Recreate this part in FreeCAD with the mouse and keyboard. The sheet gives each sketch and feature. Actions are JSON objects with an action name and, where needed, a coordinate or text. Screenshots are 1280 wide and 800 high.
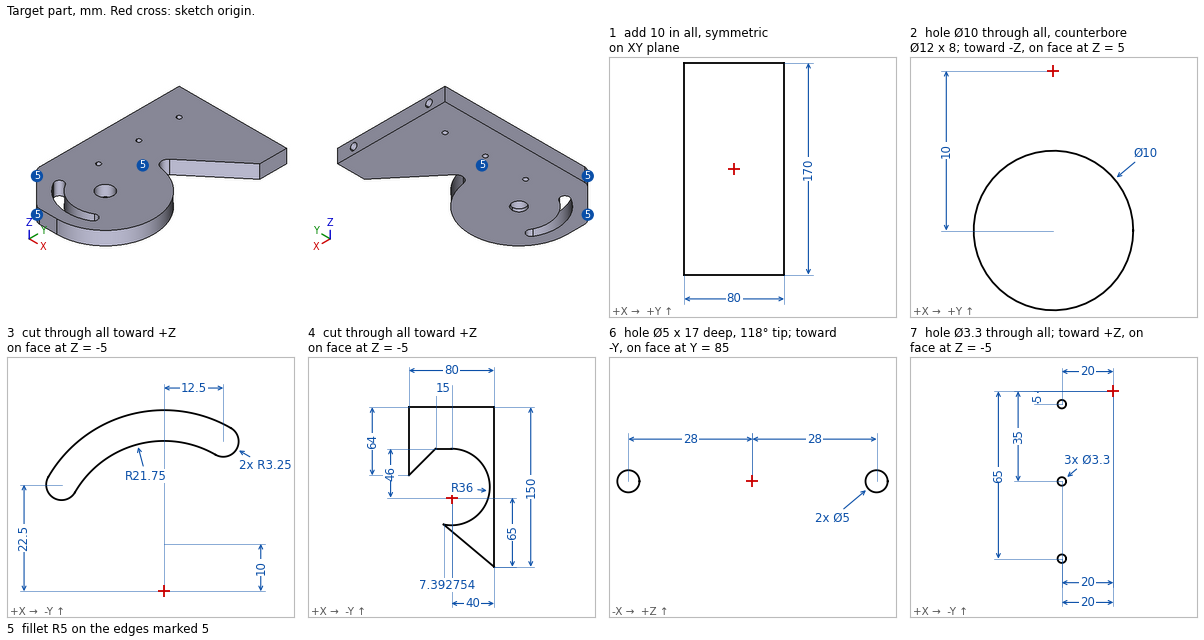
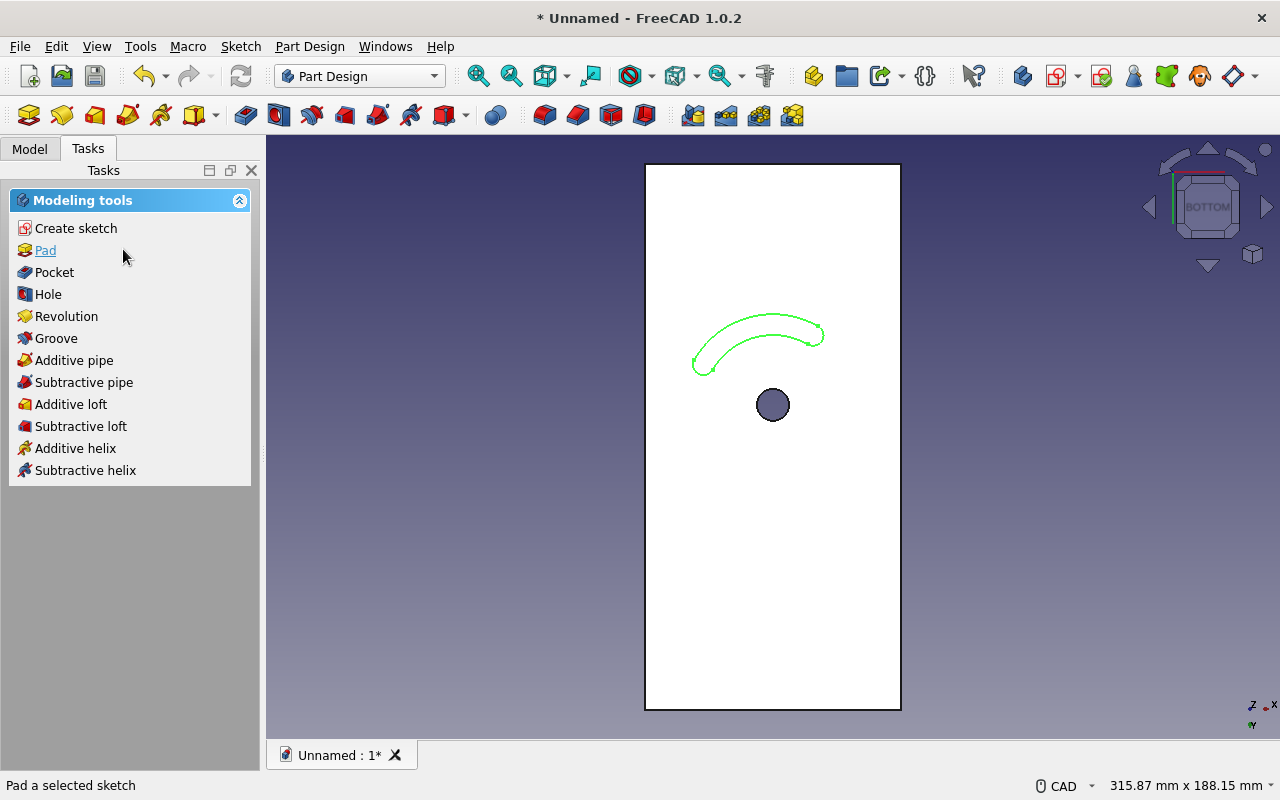
{"action": "left_click", "coordinate": [246, 116]}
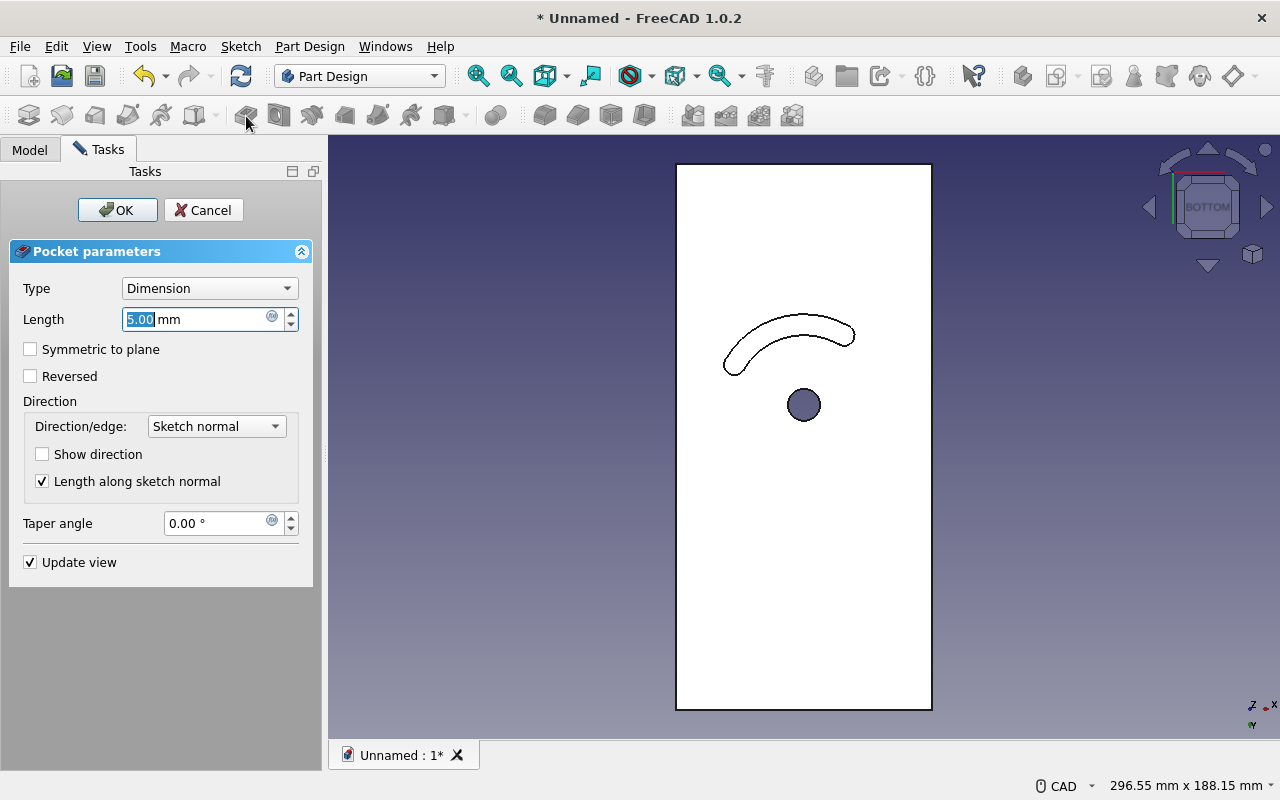
{"action": "left_click", "coordinate": [210, 288]}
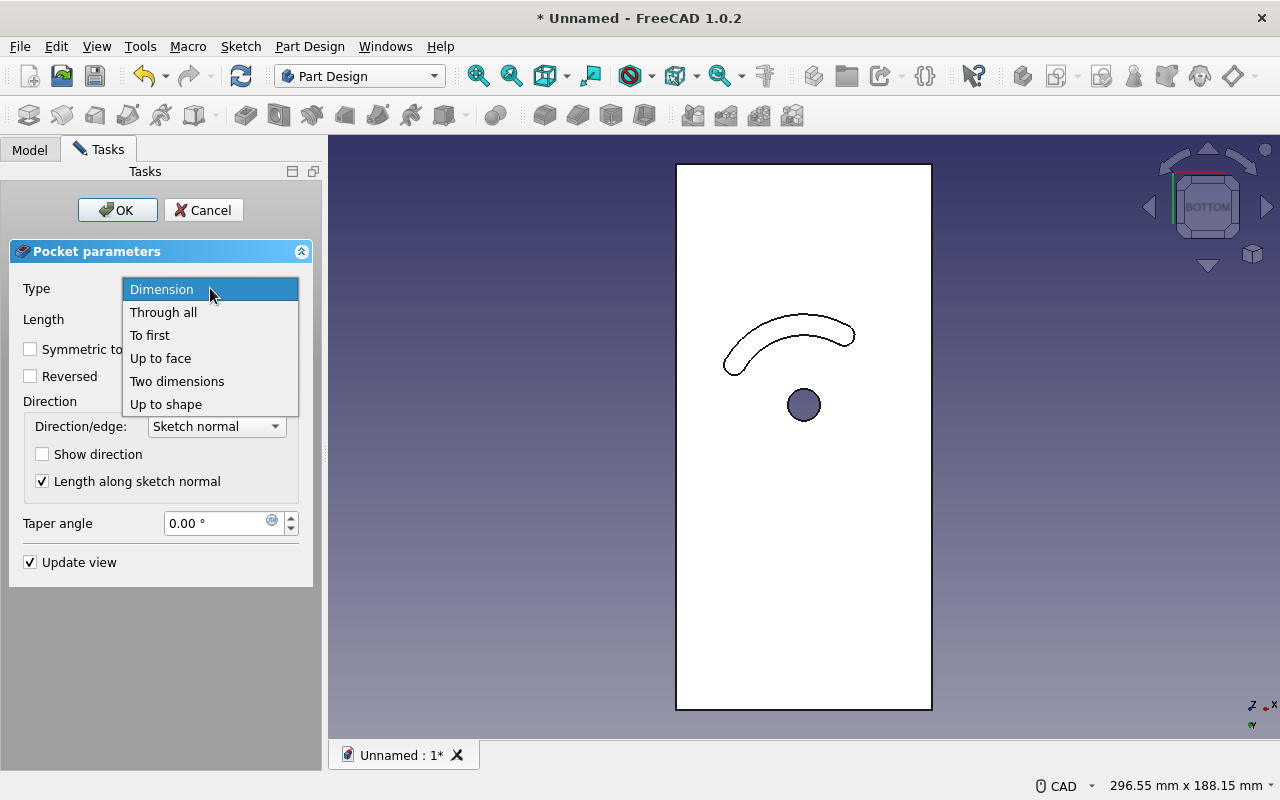
{"action": "left_click", "coordinate": [208, 312]}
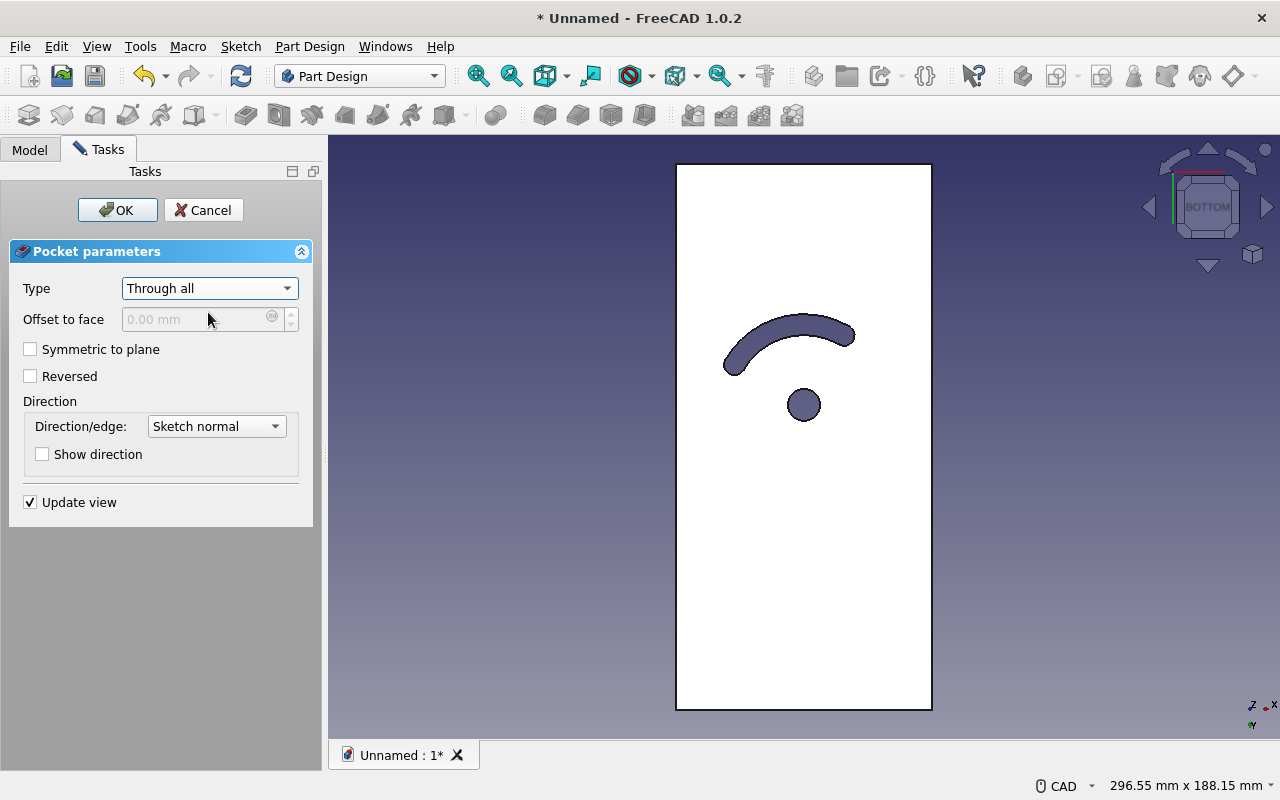
{"action": "left_click", "coordinate": [118, 210]}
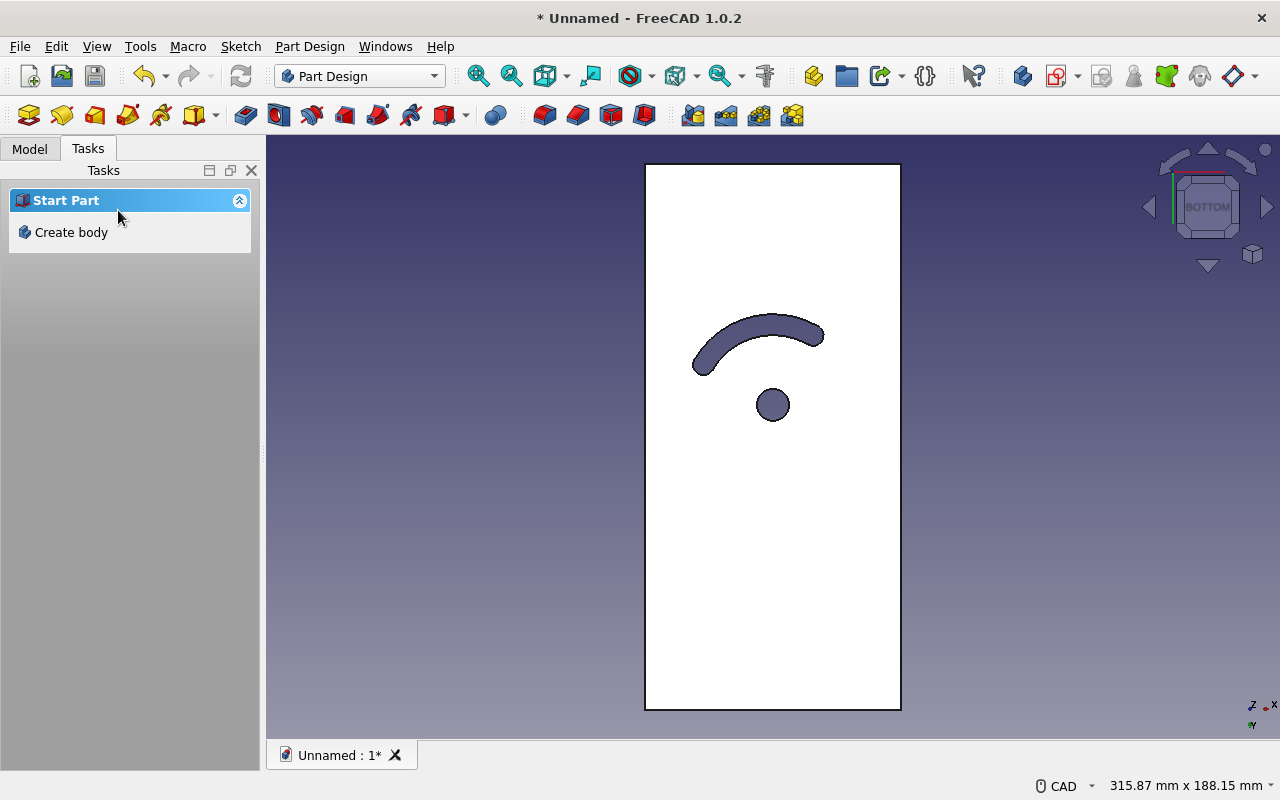
{"action": "left_click", "coordinate": [773, 592]}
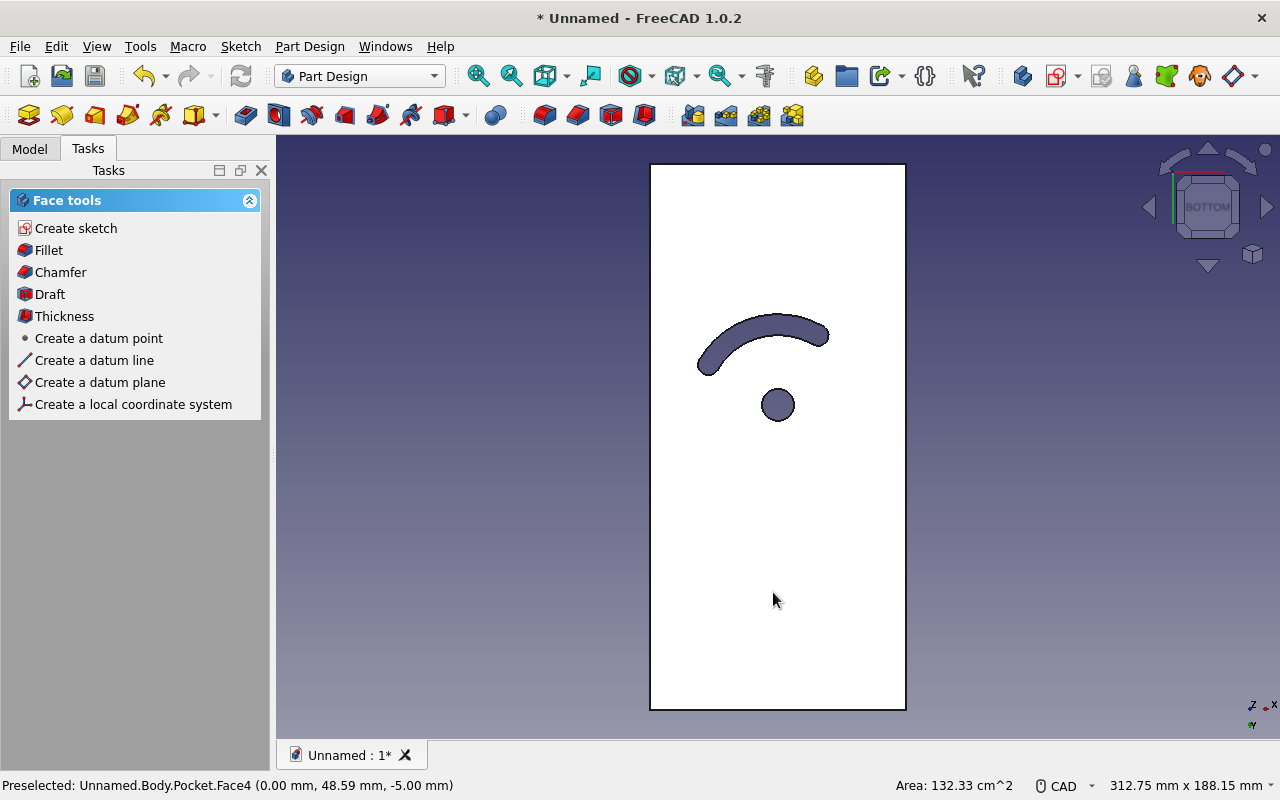
{"action": "left_click", "coordinate": [1056, 76]}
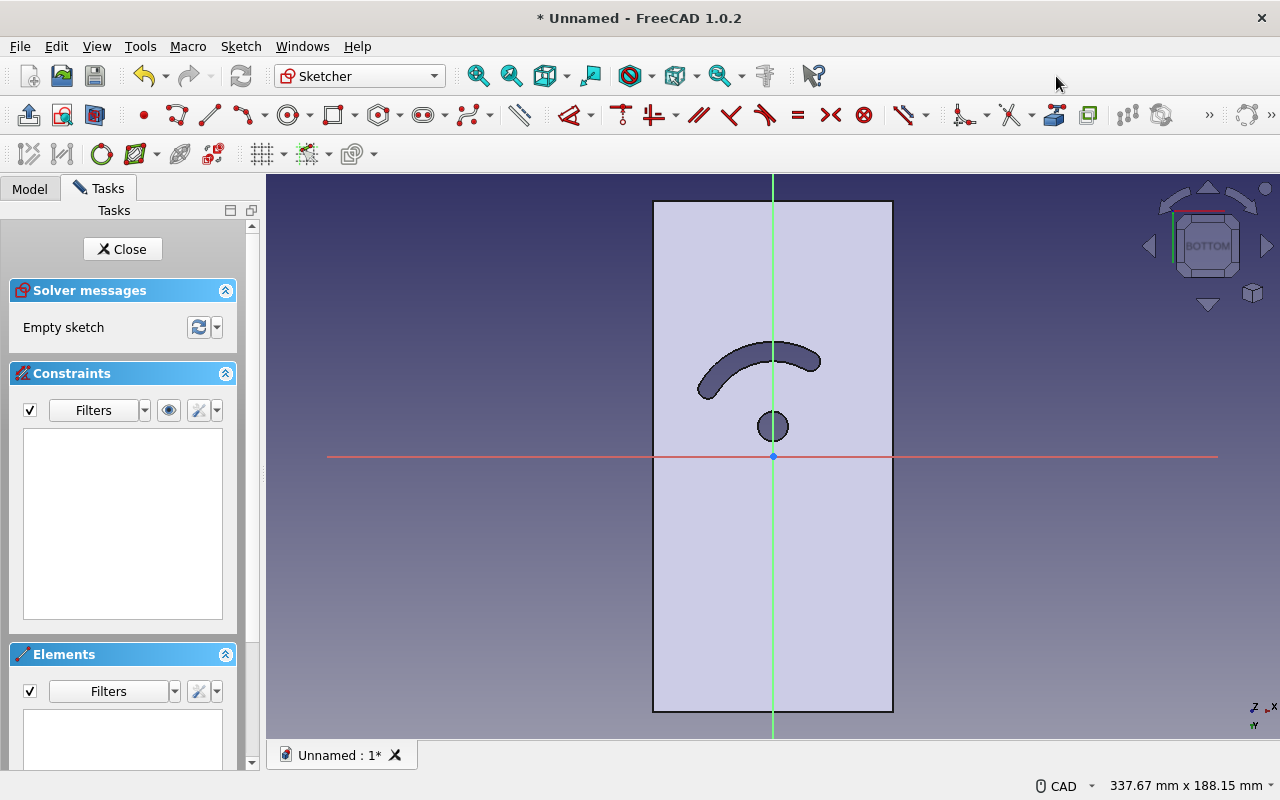
{"action": "scroll", "coordinate": [395, 592], "scroll_direction": "down", "scroll_amount": 1}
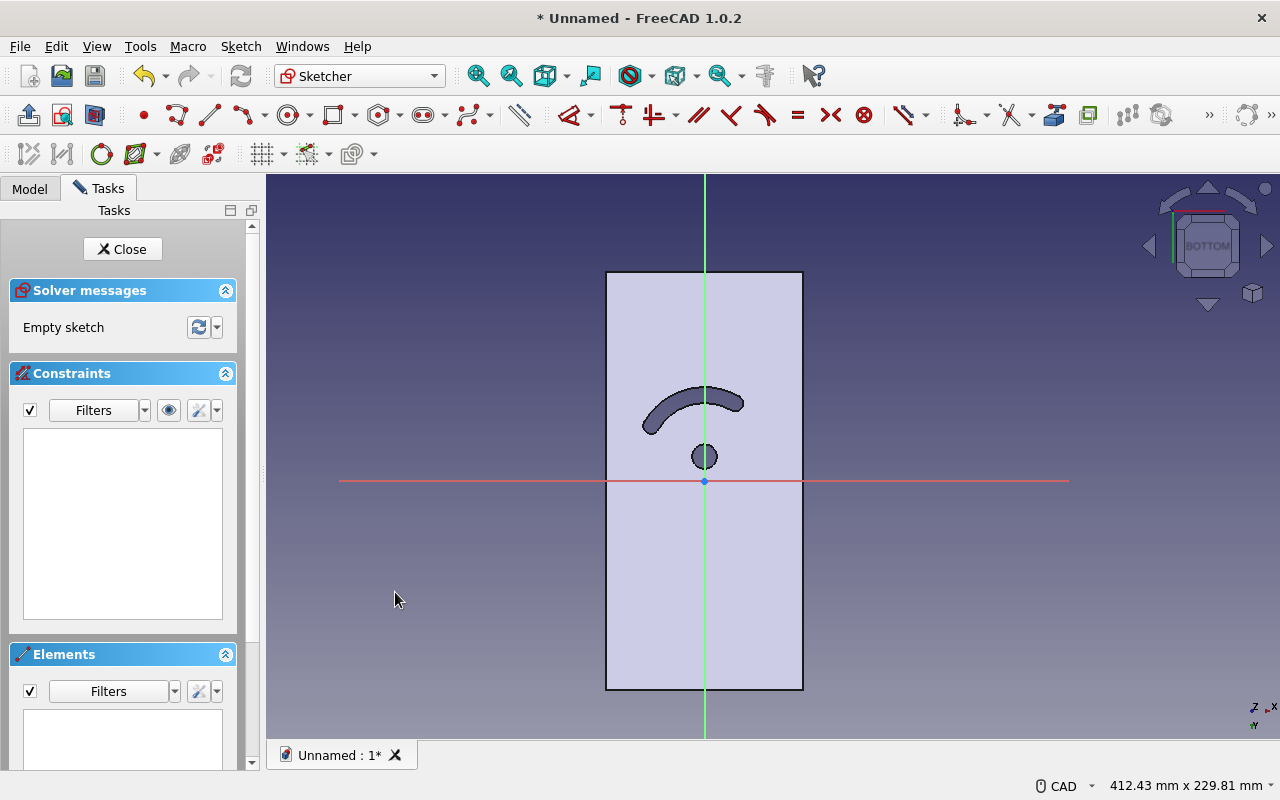
{"action": "left_click", "coordinate": [177, 116]}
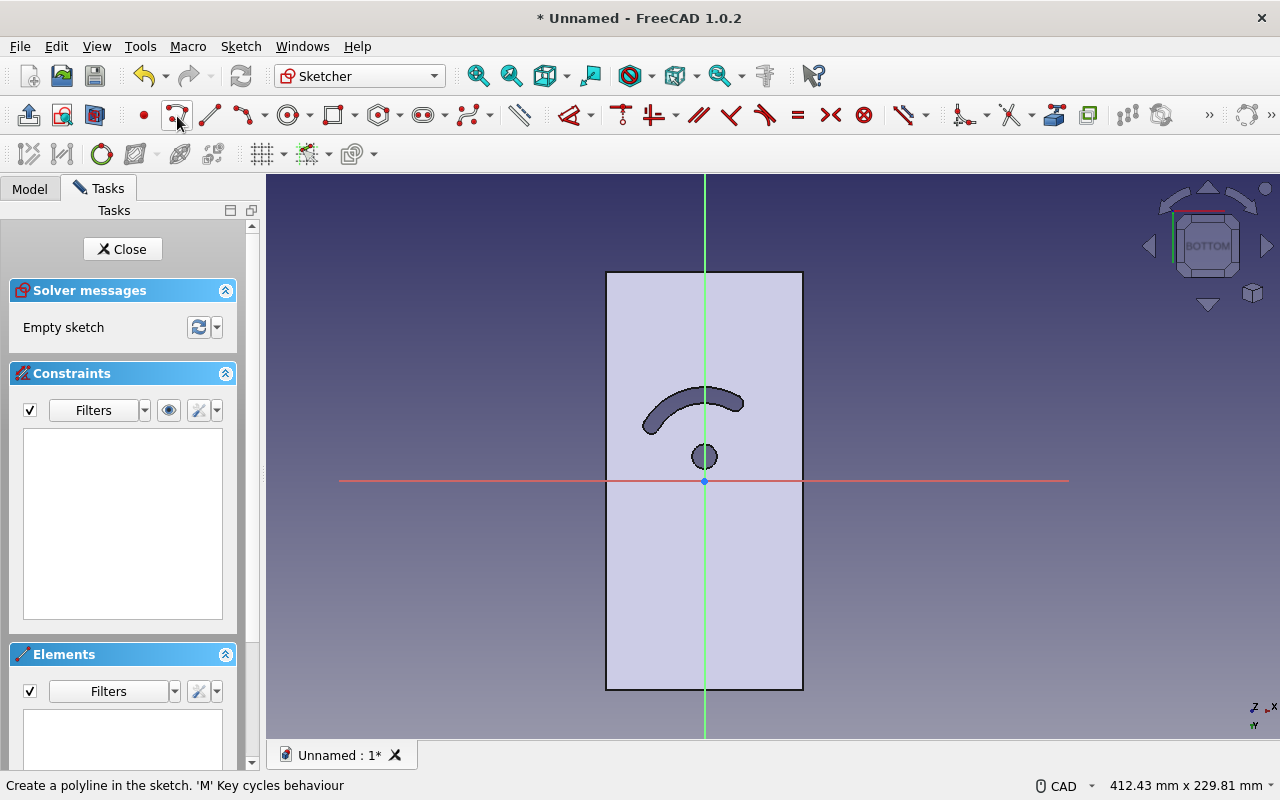
{"action": "left_click", "coordinate": [686, 543]}
{"action": "left_click", "coordinate": [803, 641]}
{"action": "left_click", "coordinate": [803, 272]}
{"action": "left_click", "coordinate": [606, 272]}
{"action": "left_click", "coordinate": [606, 430]}
{"action": "left_click", "coordinate": [668, 368]}
{"action": "left_click", "coordinate": [705, 368]}
{"action": "right_click", "coordinate": [705, 368]}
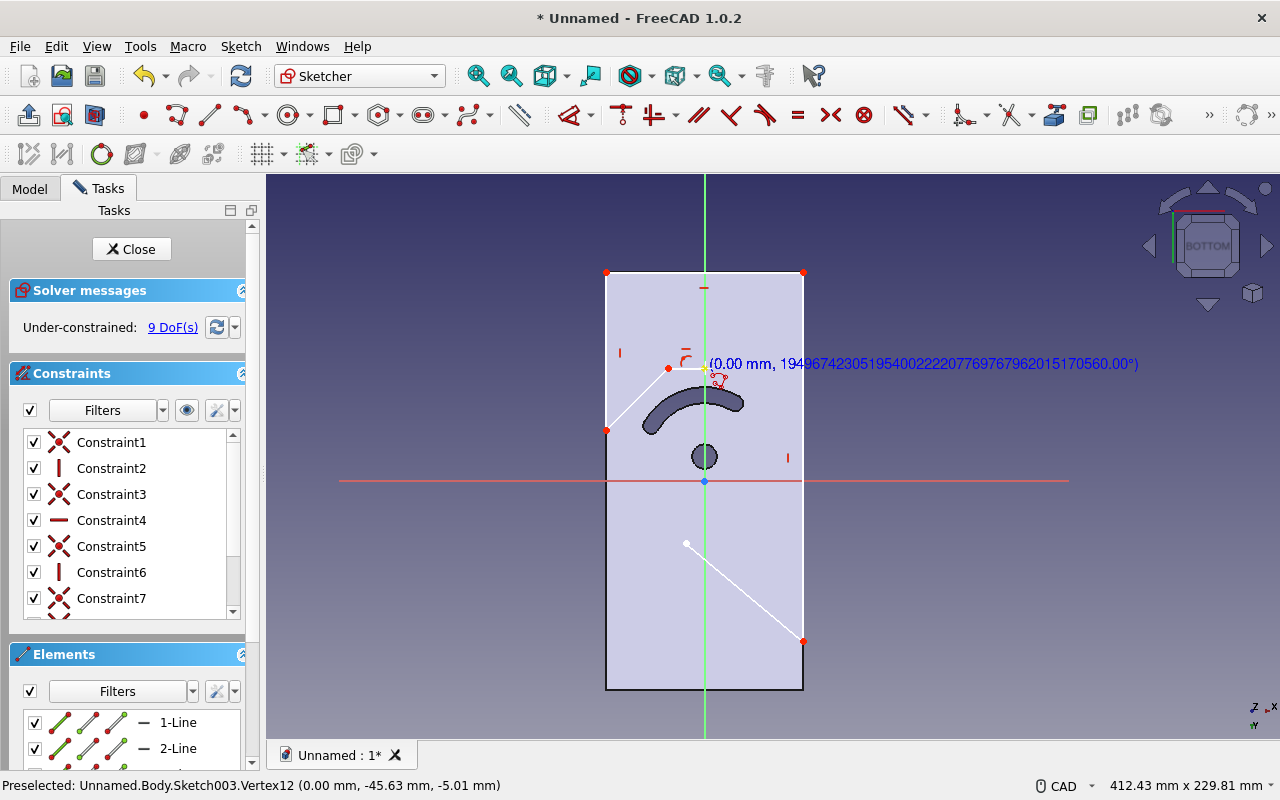
{"action": "left_click", "coordinate": [242, 116]}